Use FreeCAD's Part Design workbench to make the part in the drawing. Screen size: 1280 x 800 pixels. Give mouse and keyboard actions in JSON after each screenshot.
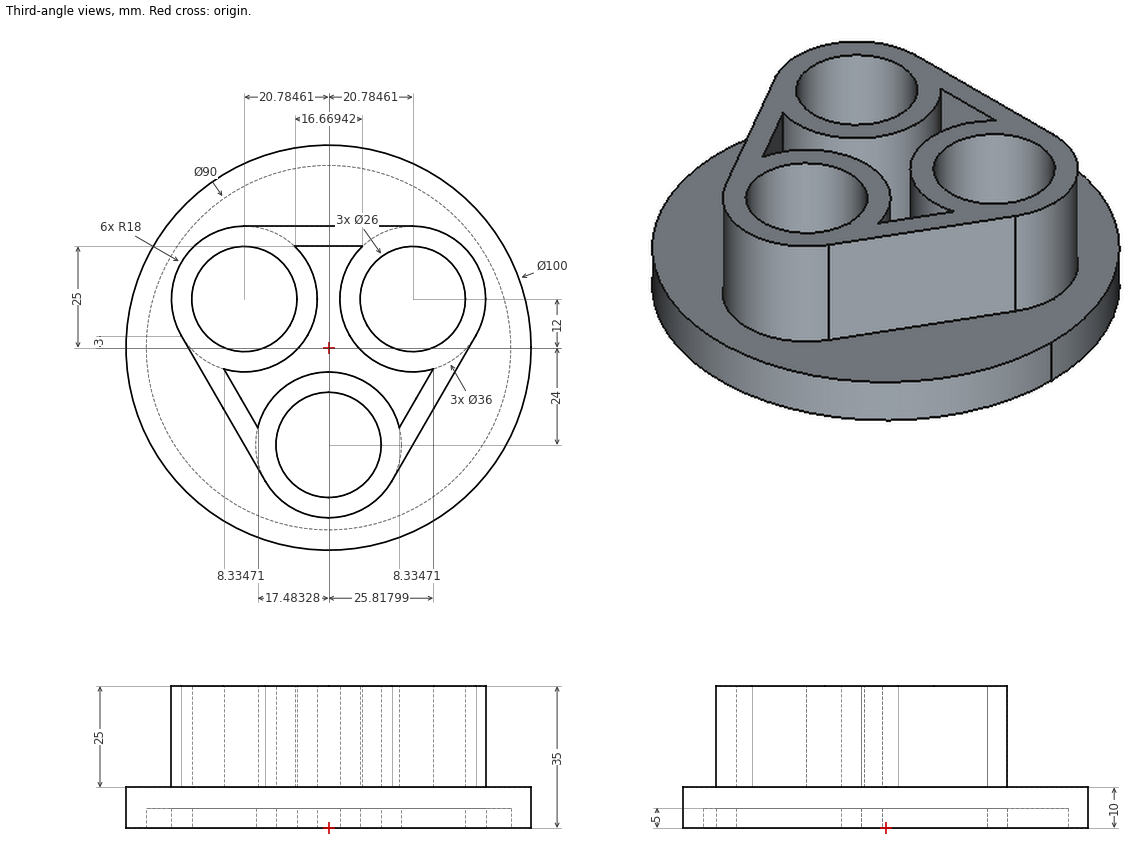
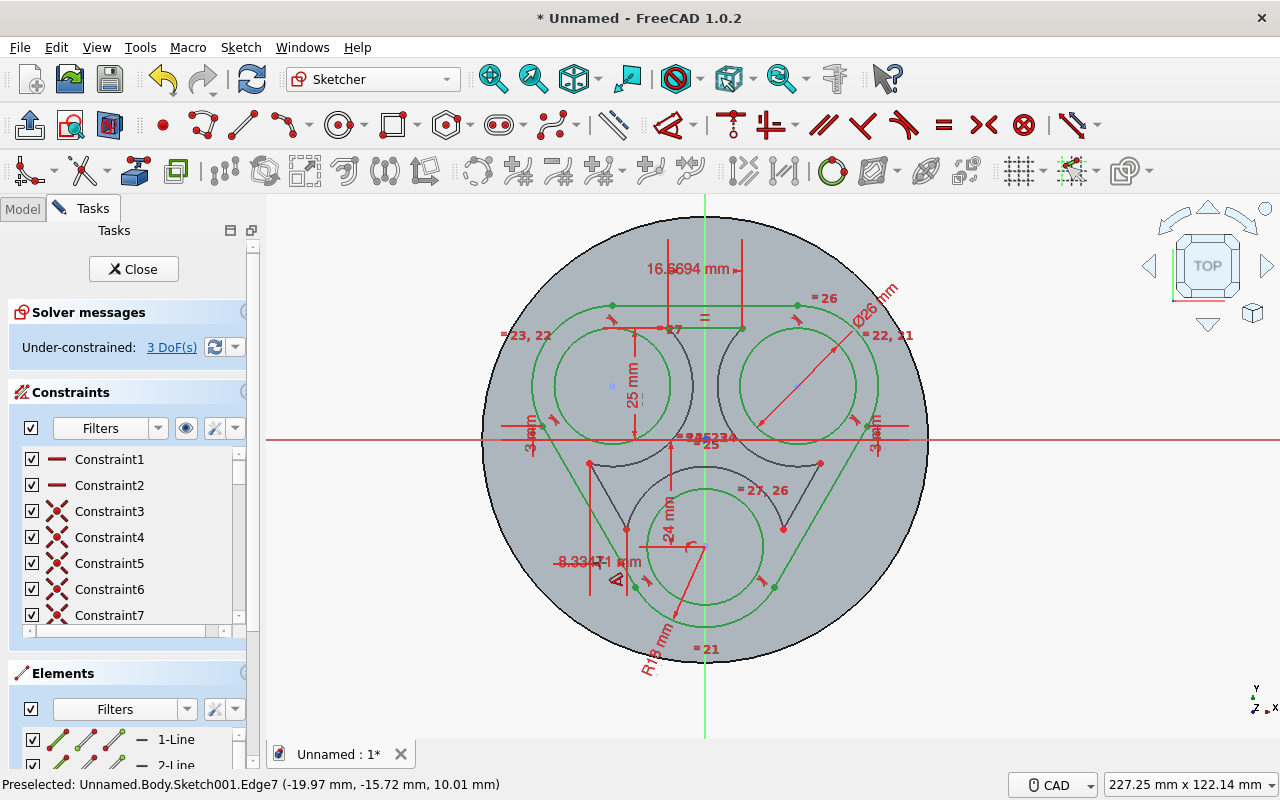
{"action": "left_click", "coordinate": [810, 483]}
{"action": "left_click", "coordinate": [811, 563]}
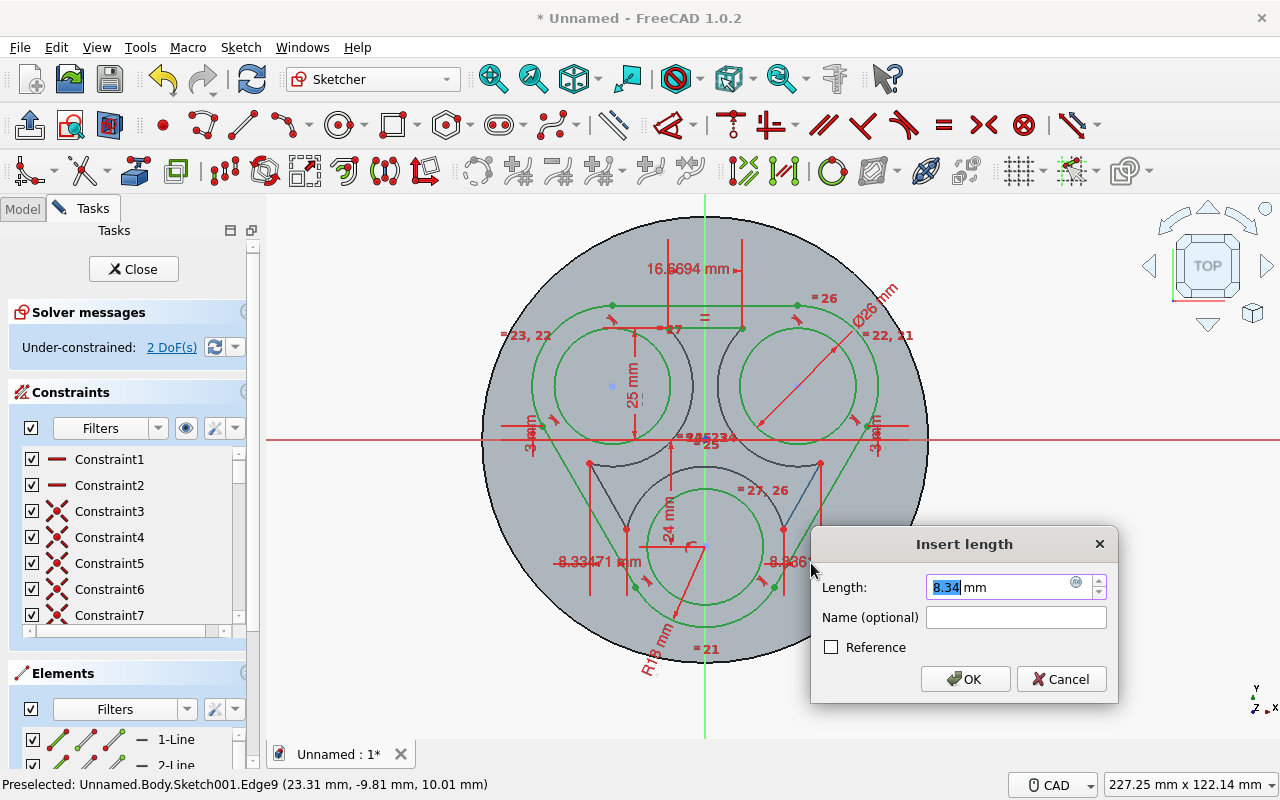
{"action": "type", "text": "8.33471"}
{"action": "key", "text": "Return"}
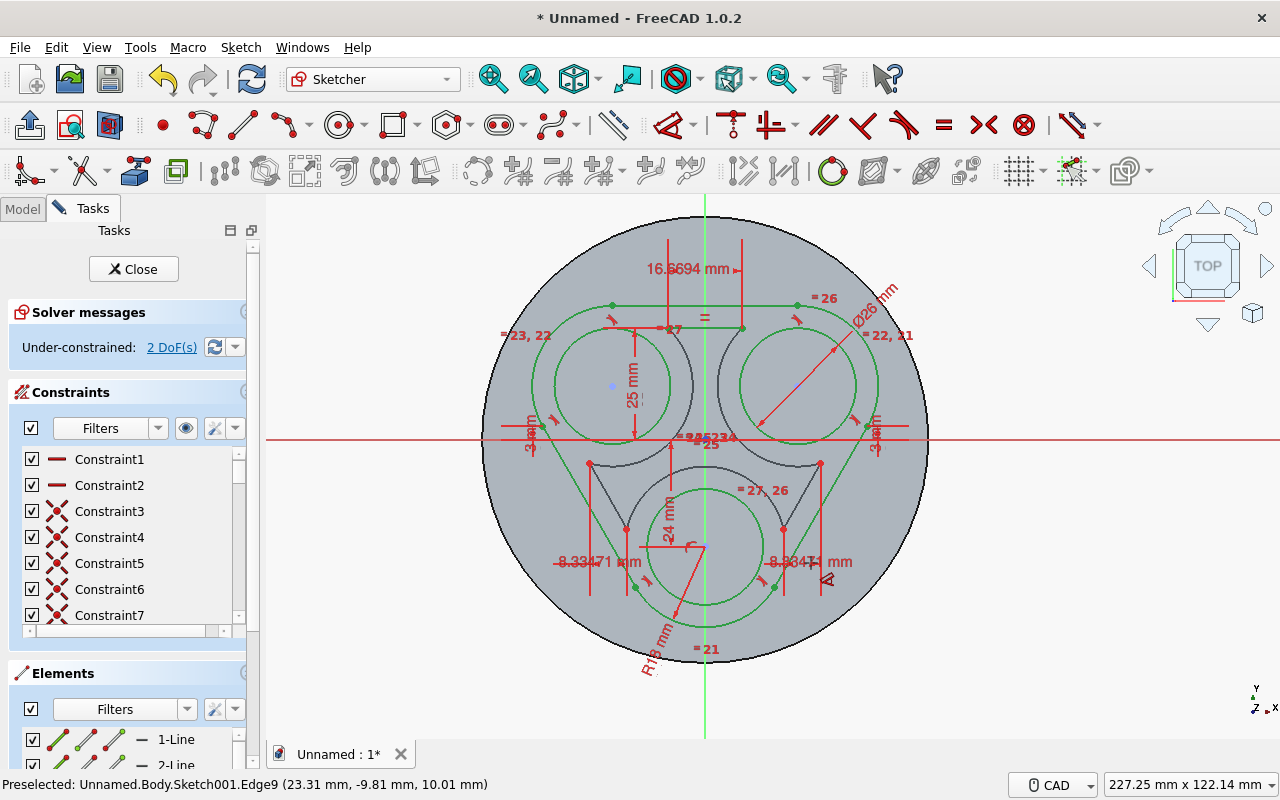
{"action": "left_click", "coordinate": [627, 529]}
{"action": "left_click", "coordinate": [684, 563]}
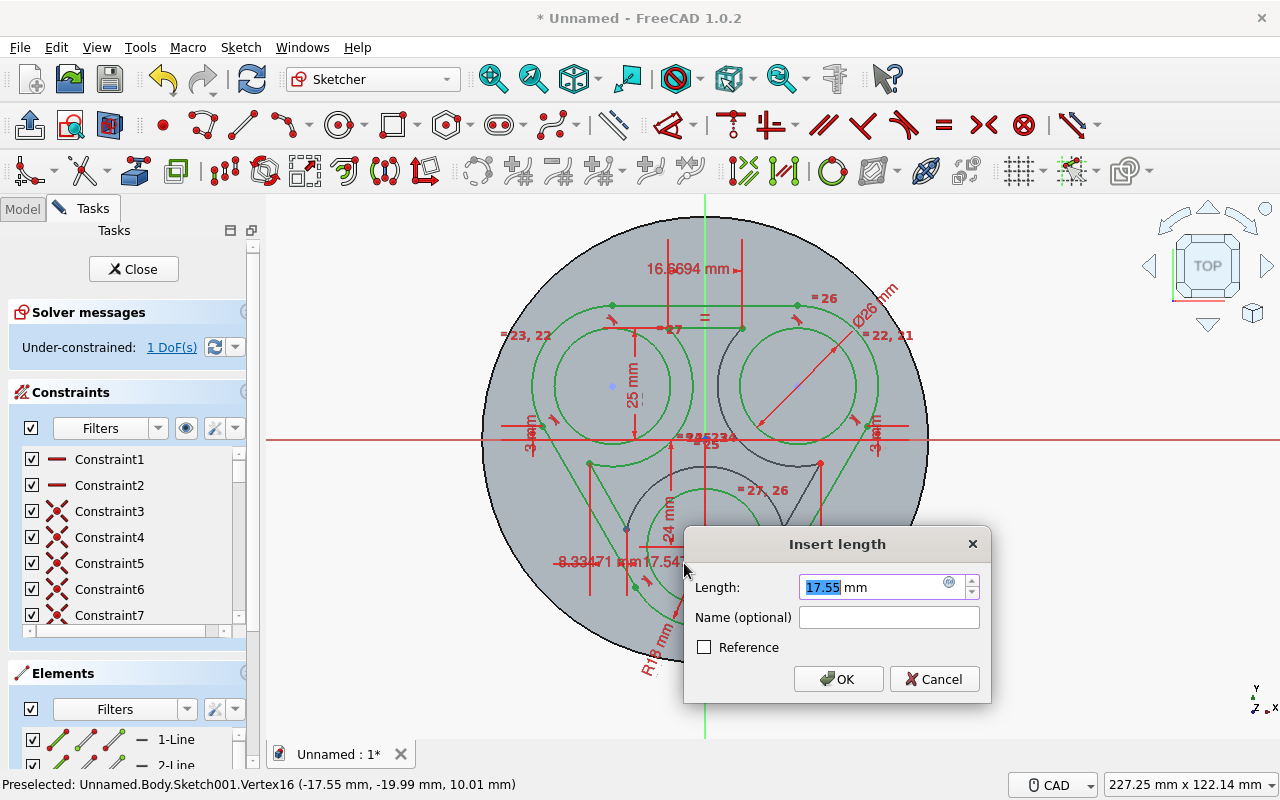
{"action": "type", "text": "17.48328"}
{"action": "key", "text": "Return"}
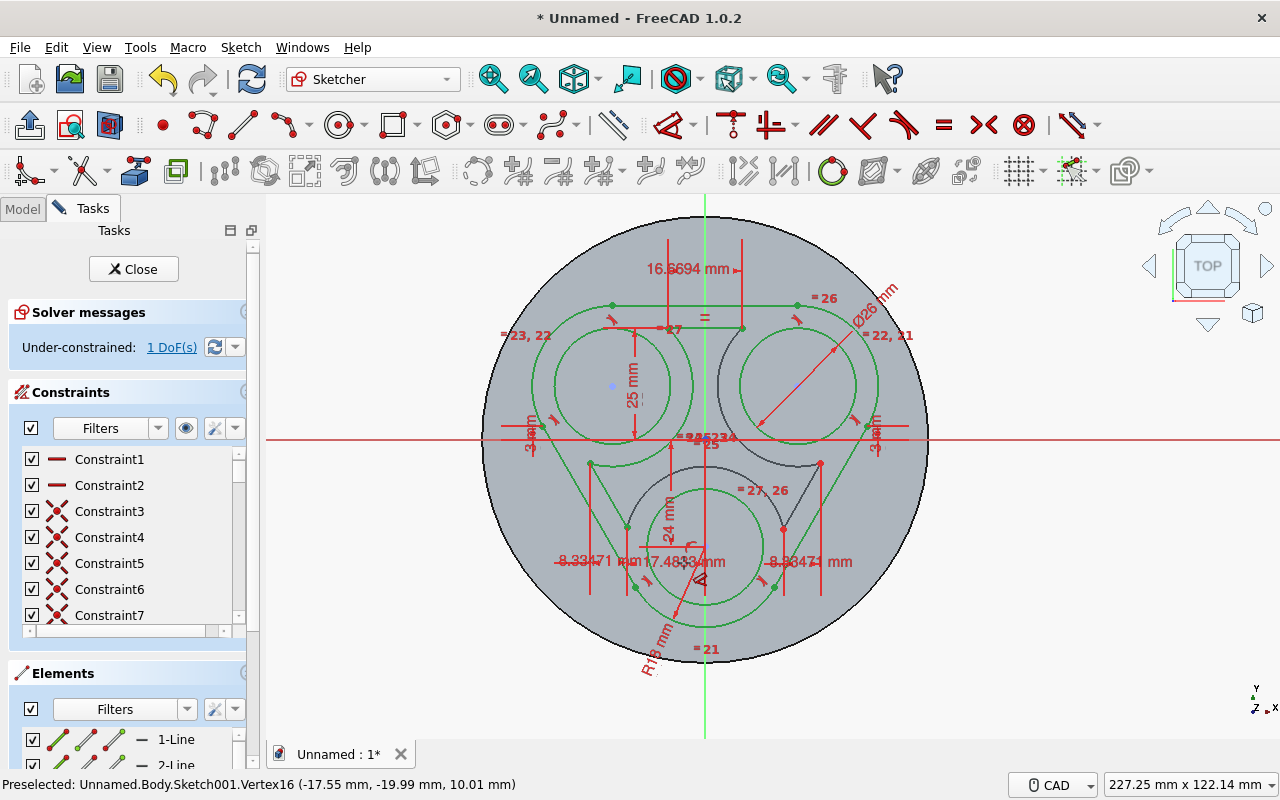
{"action": "left_click", "coordinate": [821, 463]}
{"action": "left_click", "coordinate": [763, 406]}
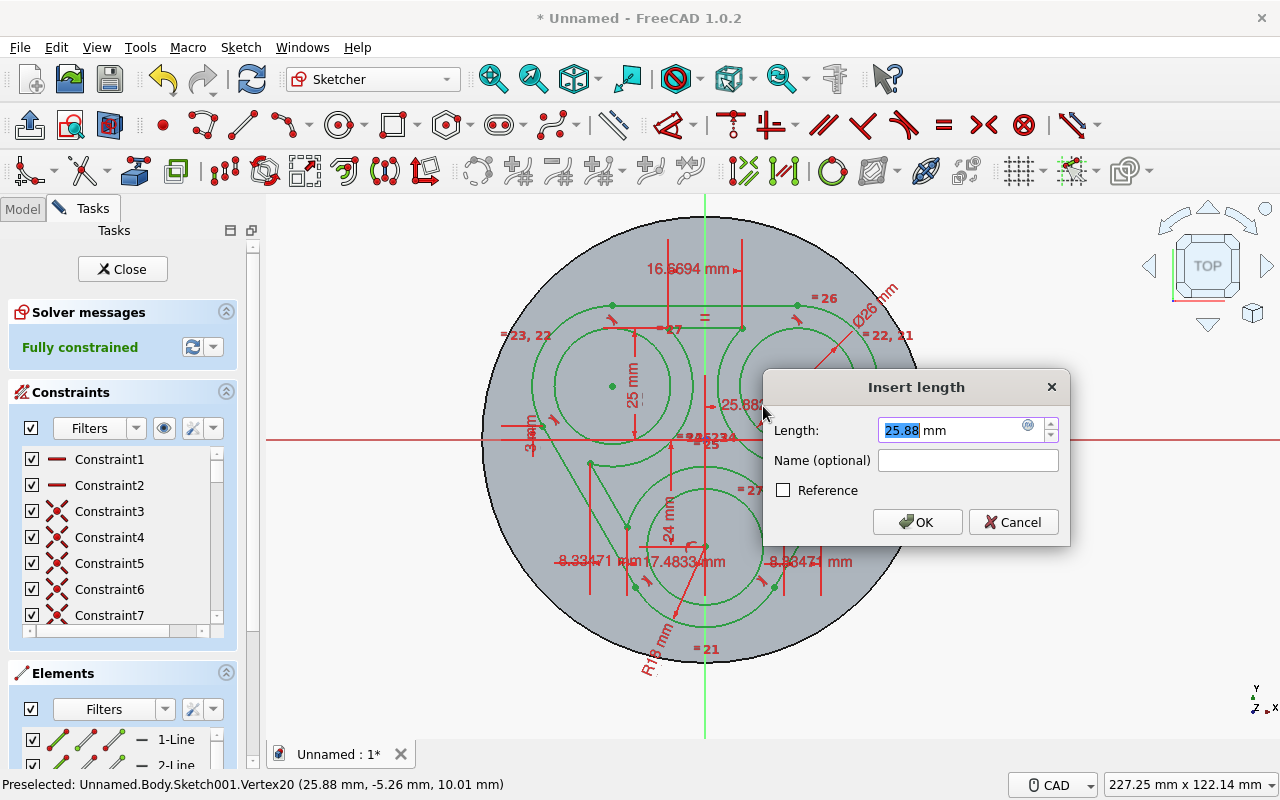
{"action": "type", "text": "25.81799"}
{"action": "key", "text": "Return"}
{"action": "key", "text": "Escape"}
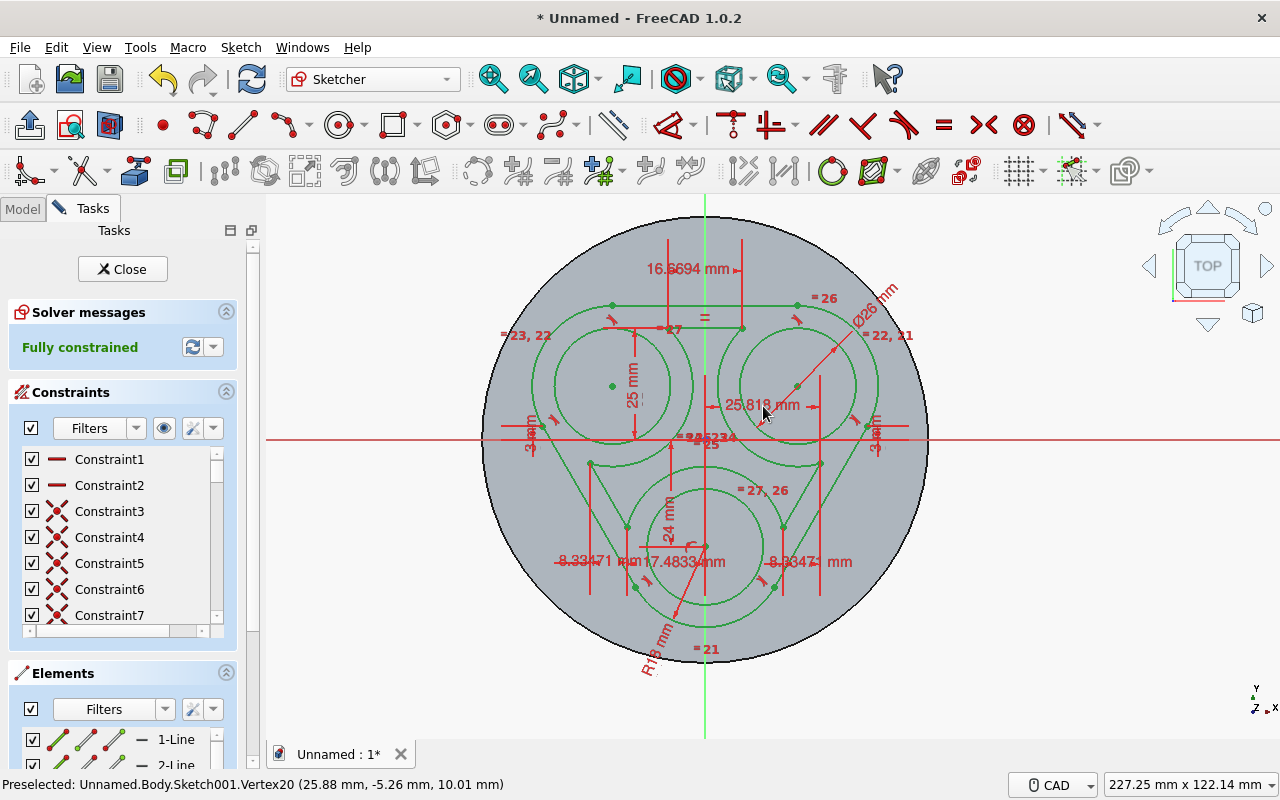
{"action": "left_click", "coordinate": [123, 269]}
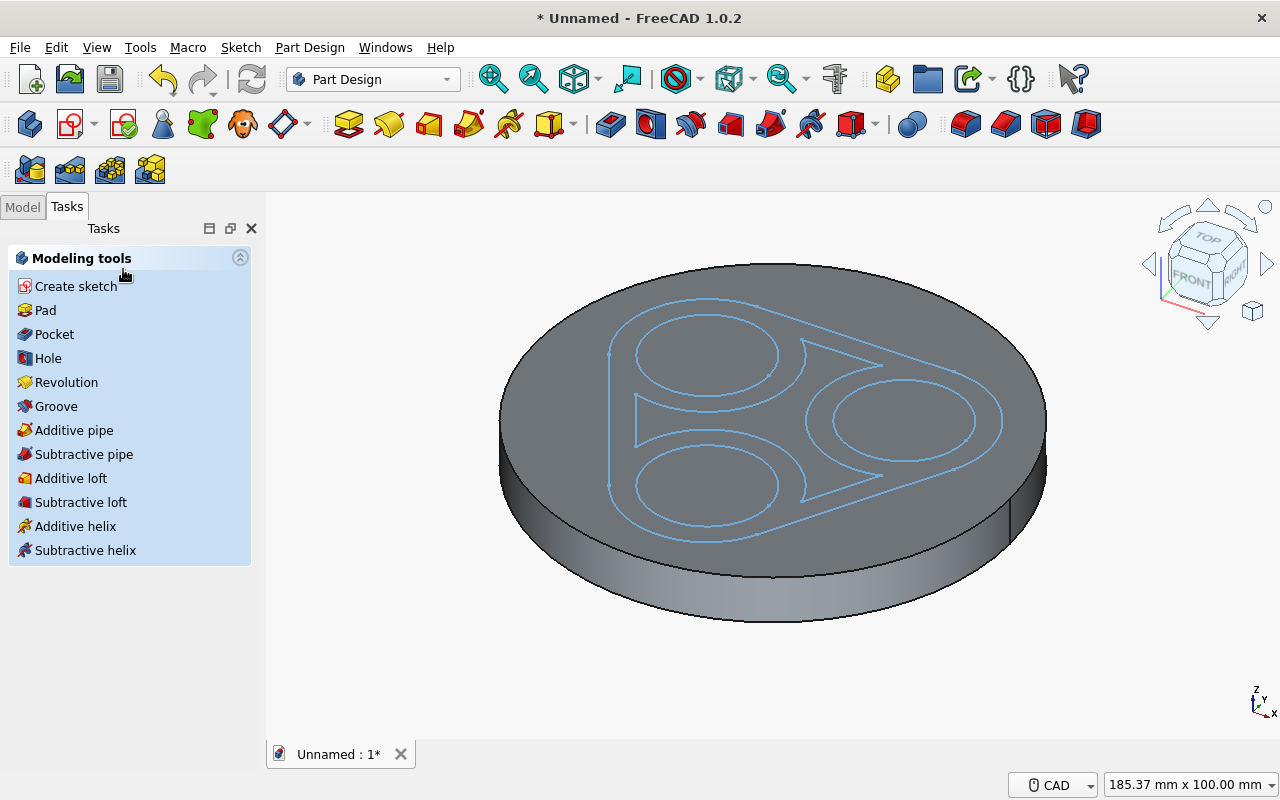
{"action": "left_click", "coordinate": [350, 124]}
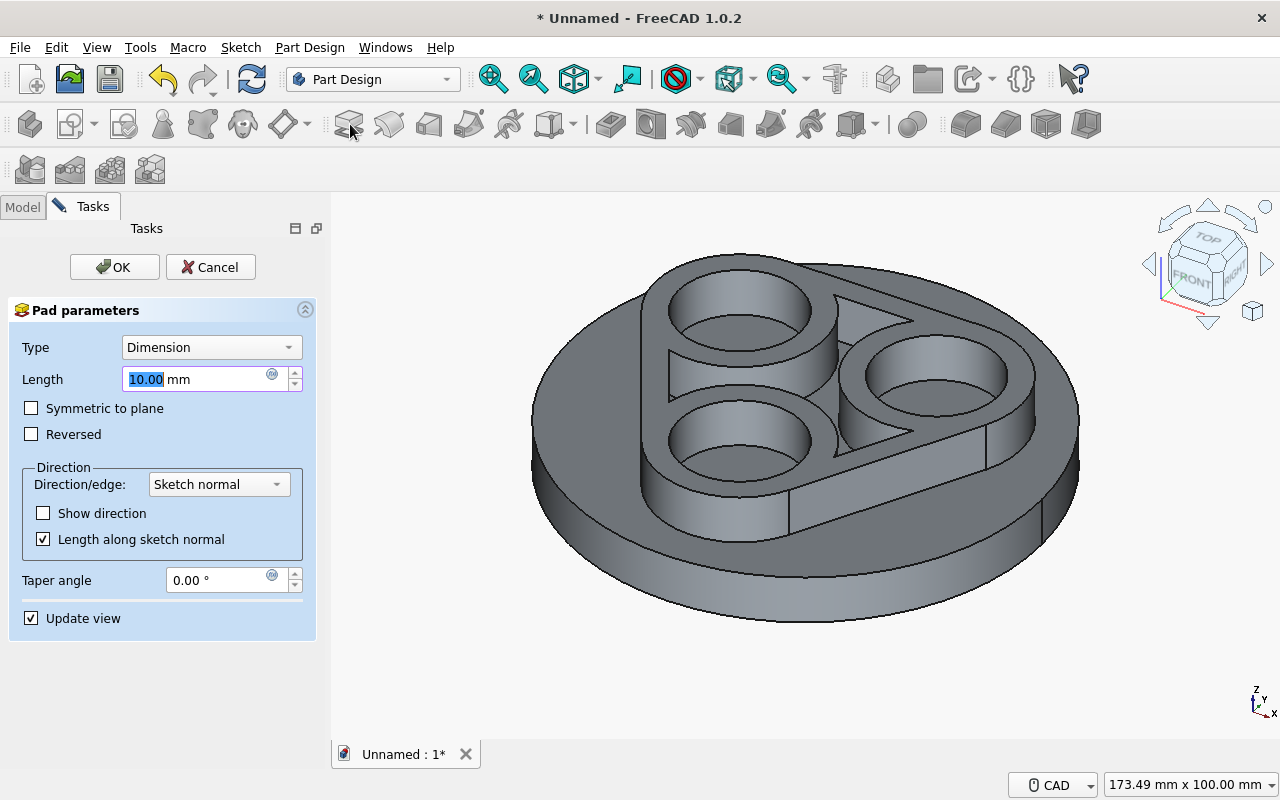
{"action": "type", "text": "25"}
{"action": "key", "text": "Tab"}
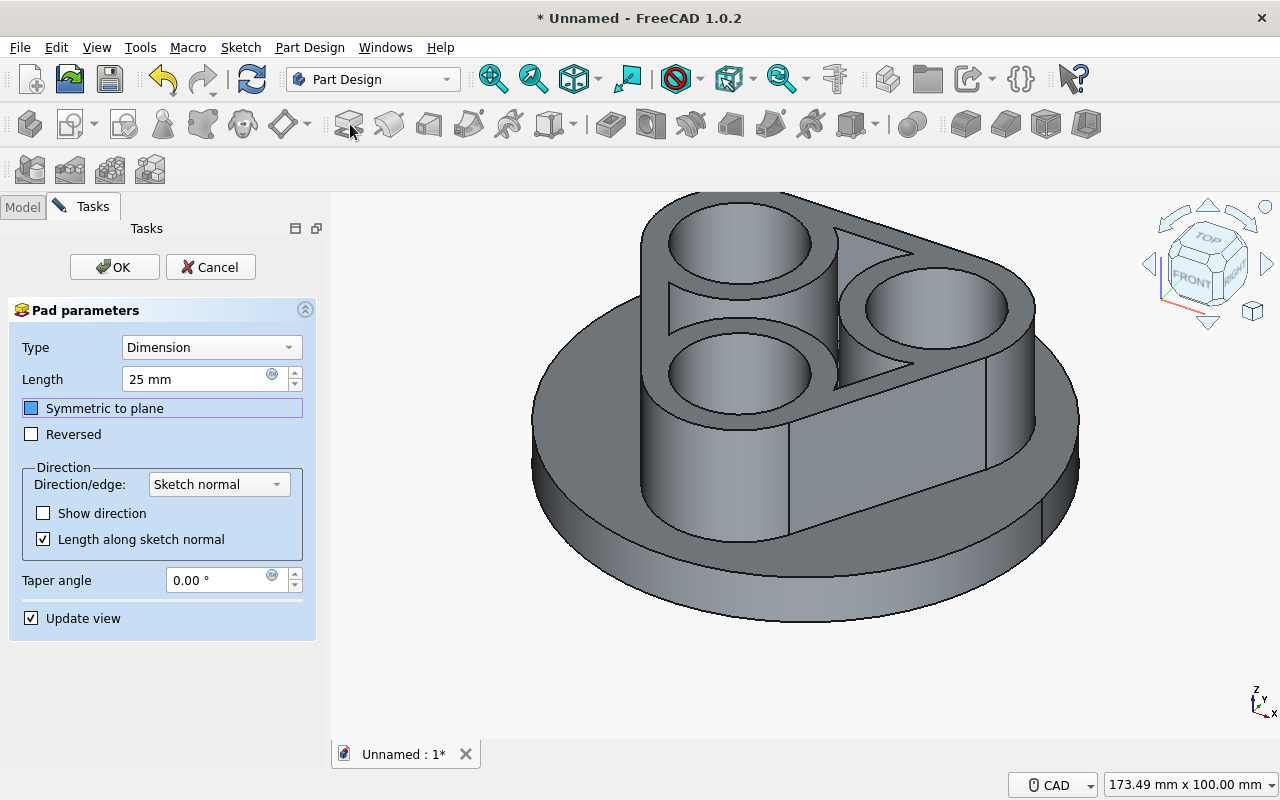
{"action": "left_click", "coordinate": [115, 267]}